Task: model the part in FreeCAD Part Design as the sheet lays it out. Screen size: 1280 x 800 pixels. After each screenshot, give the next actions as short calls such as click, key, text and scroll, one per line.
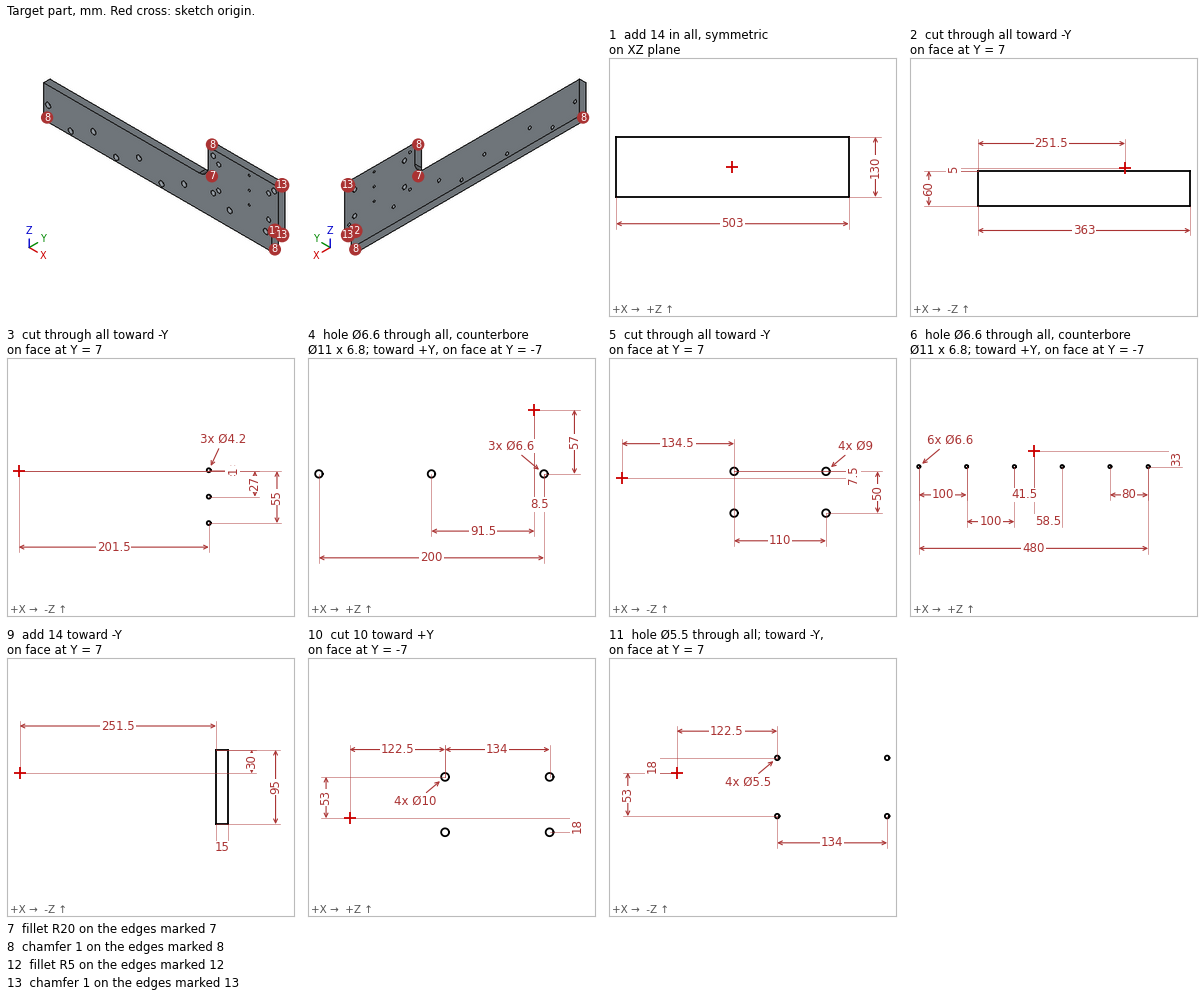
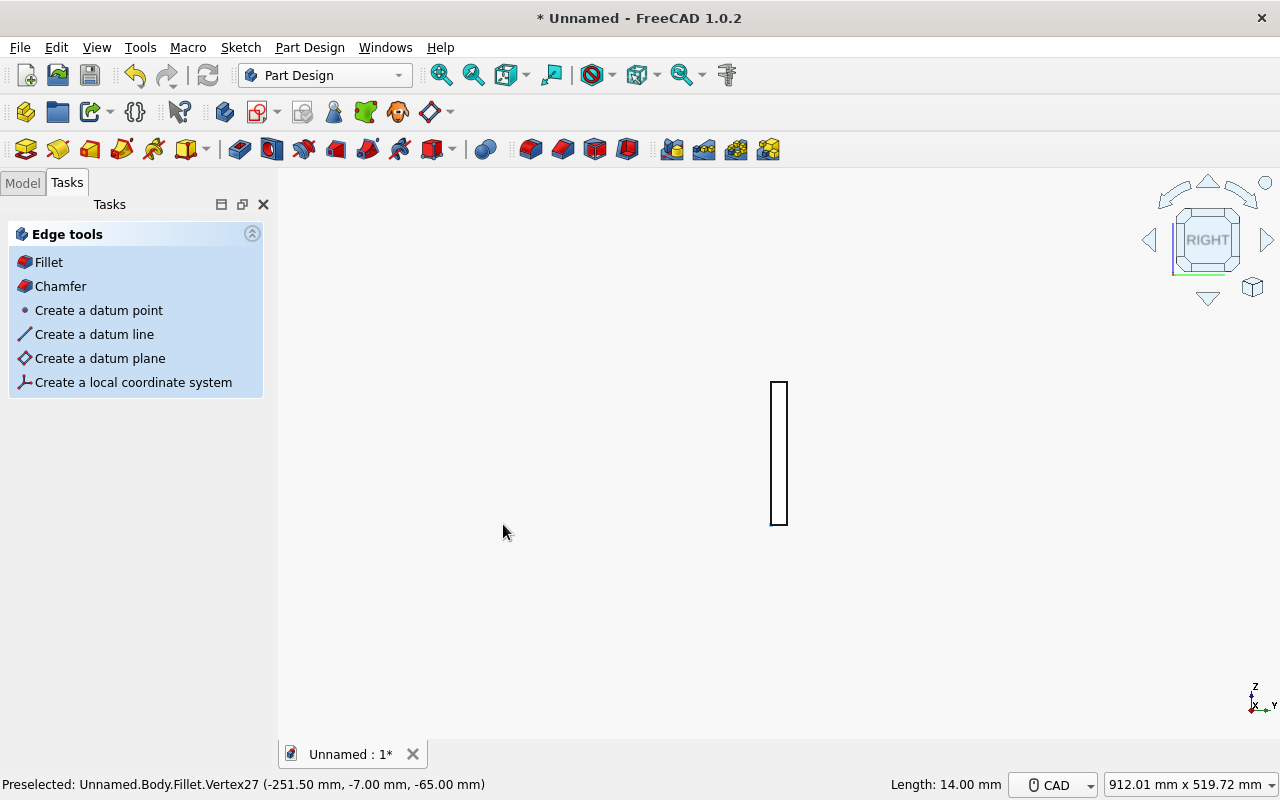
click(442, 76)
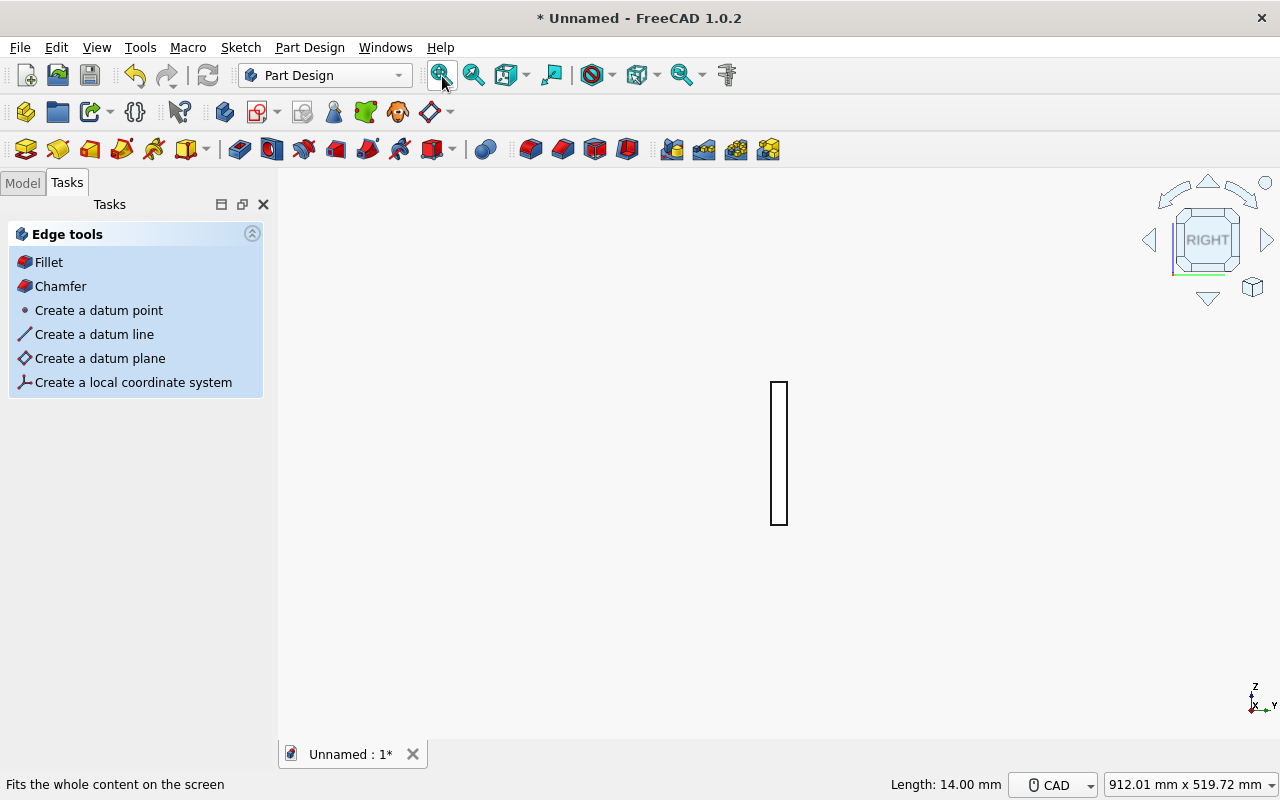
click(779, 524, ctrl)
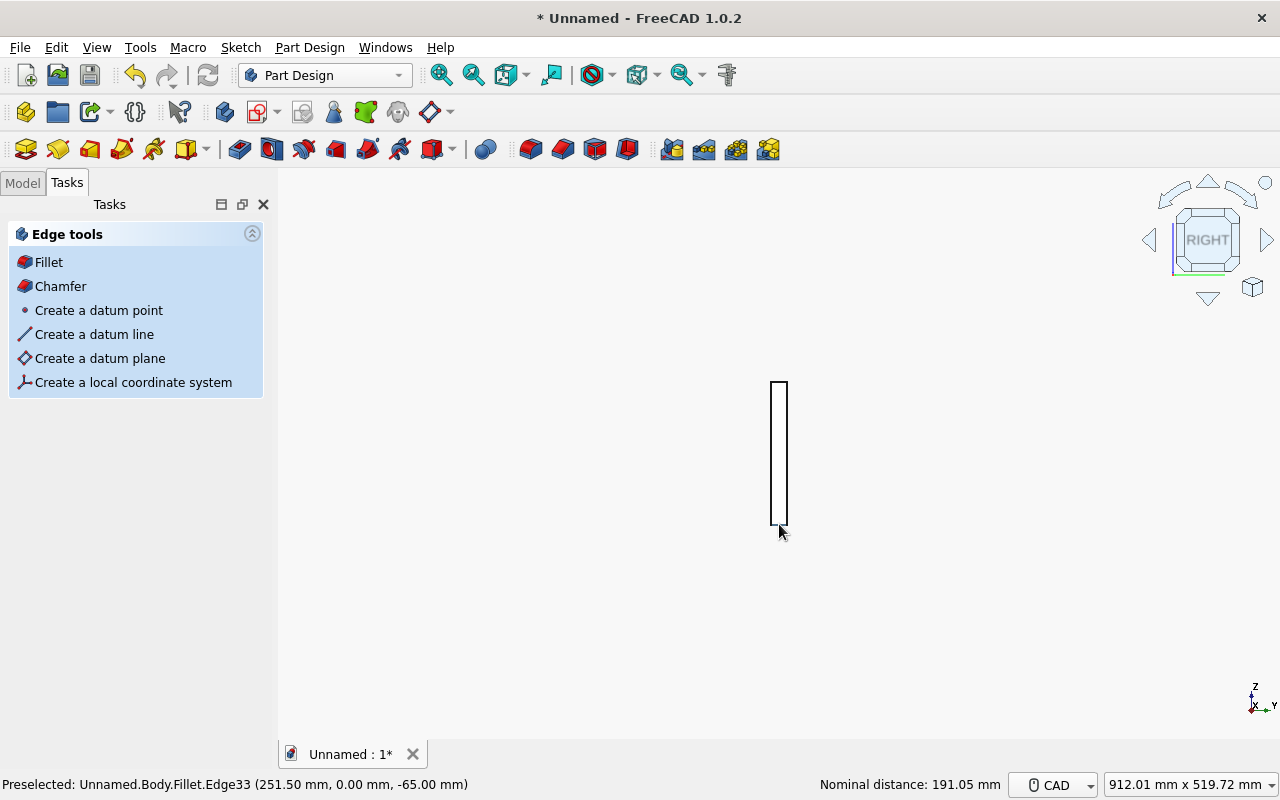
scroll(779, 524, up, 5)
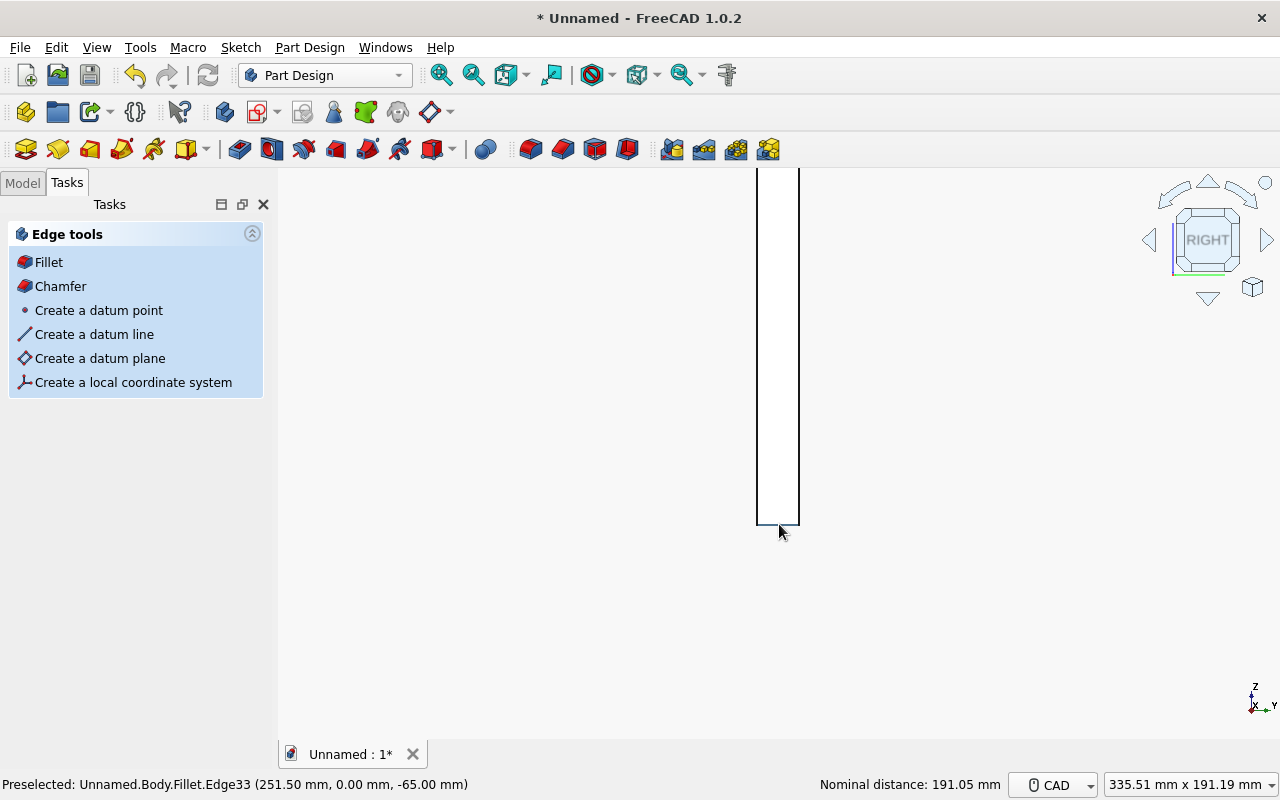
key(v)
key(f)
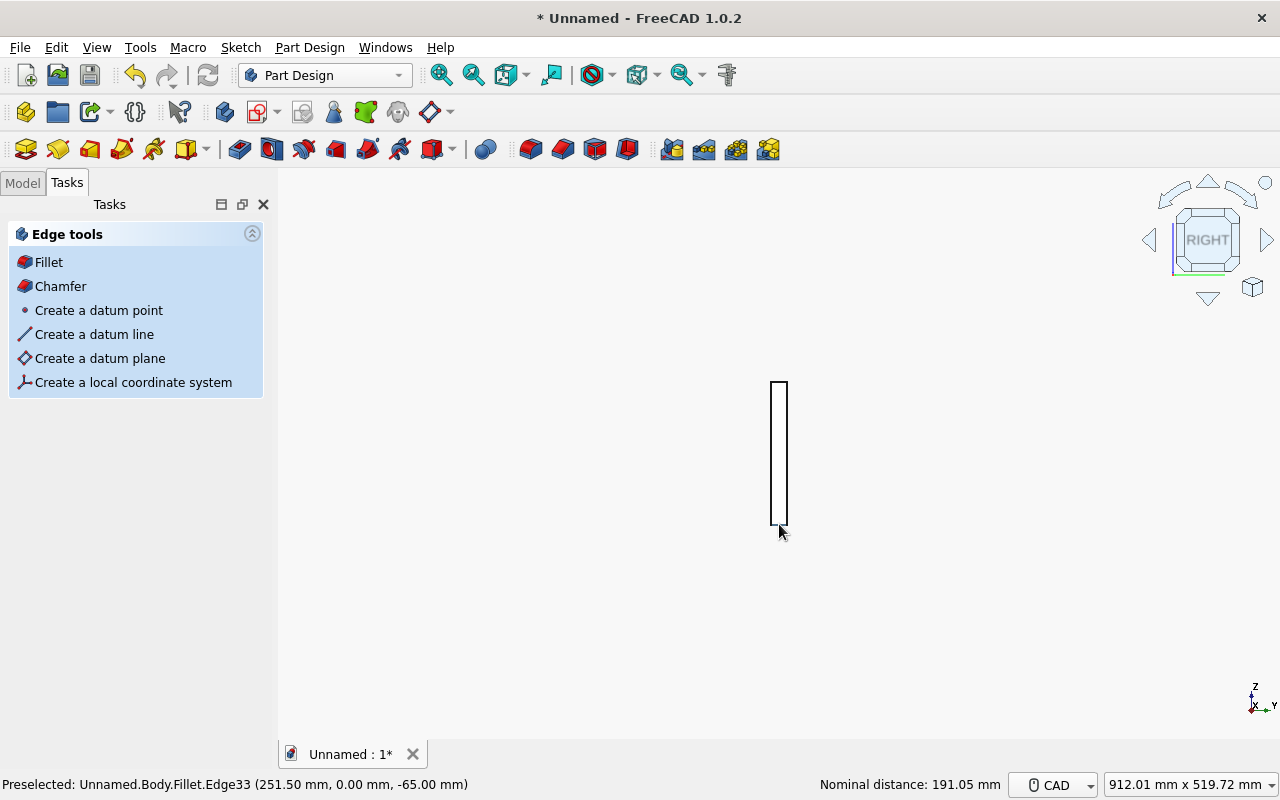
key(5)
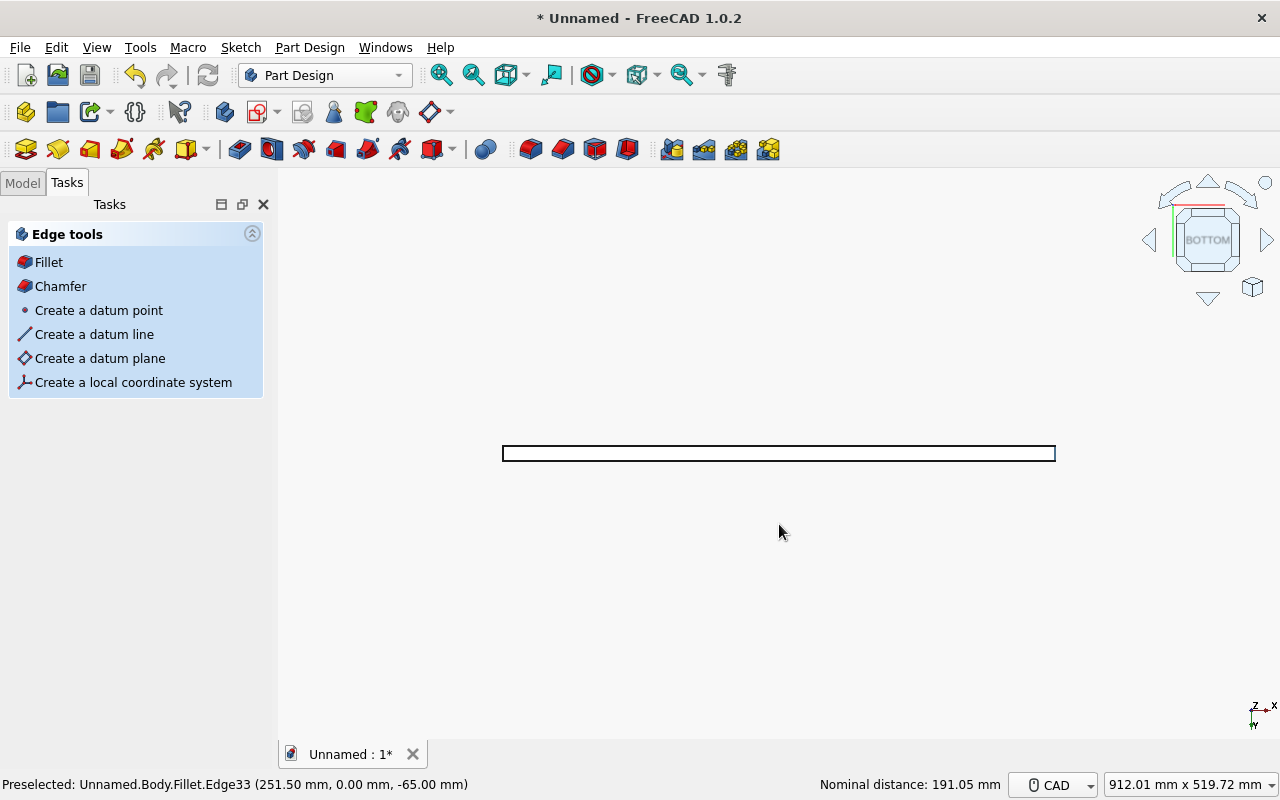
click(503, 452, ctrl)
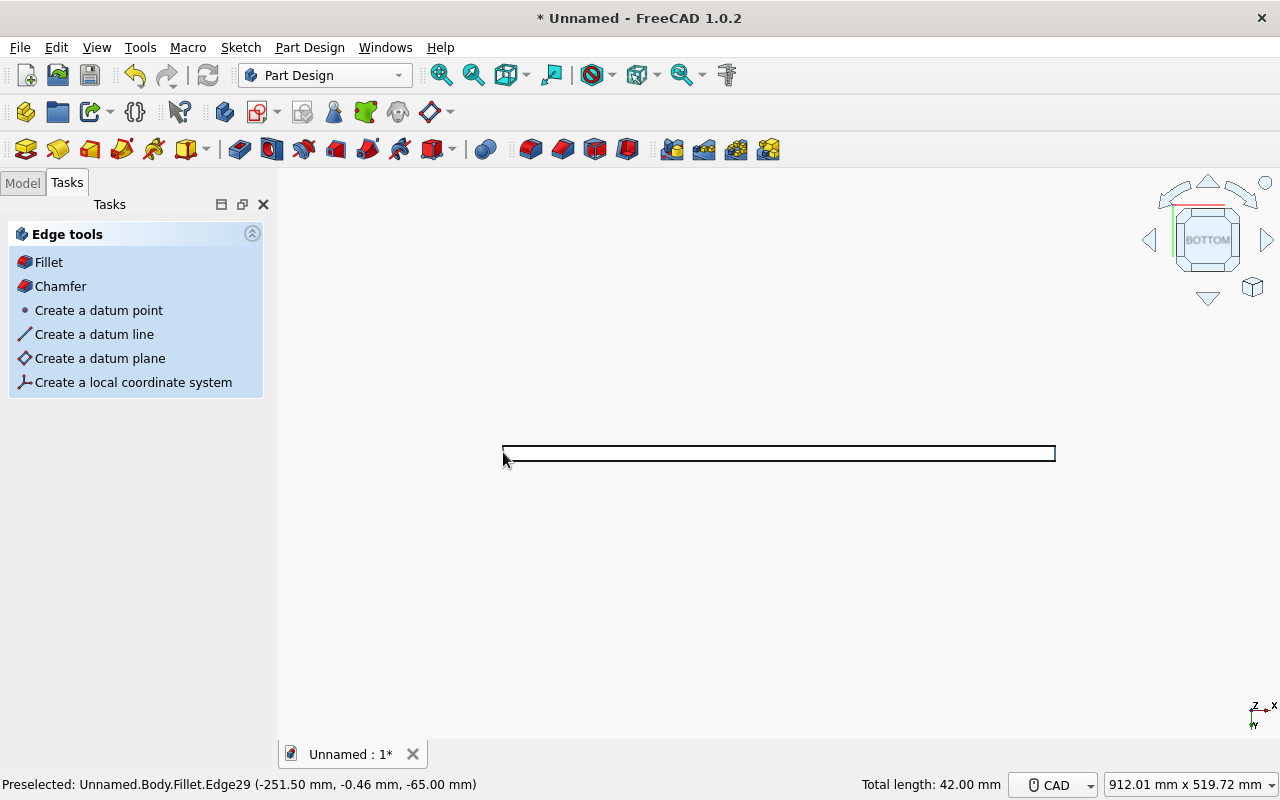
click(564, 150)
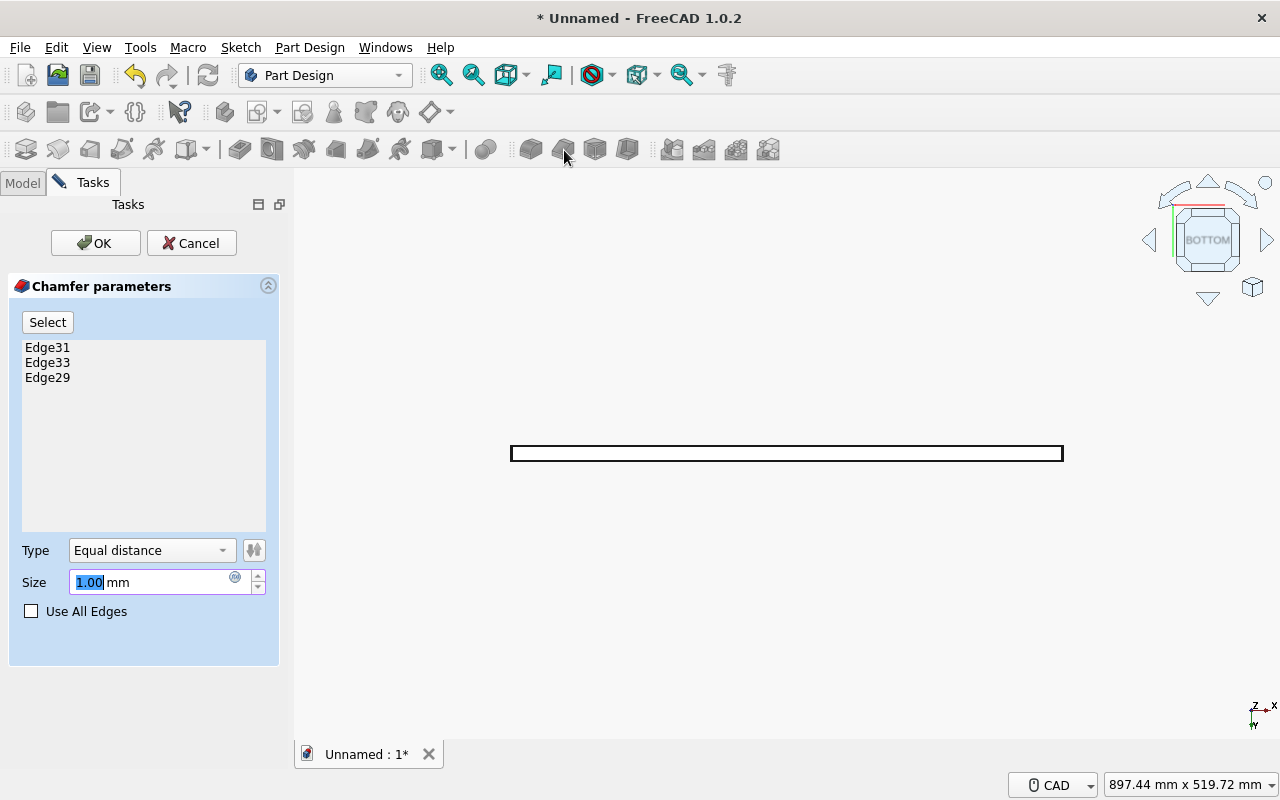
text(1)
key(Tab)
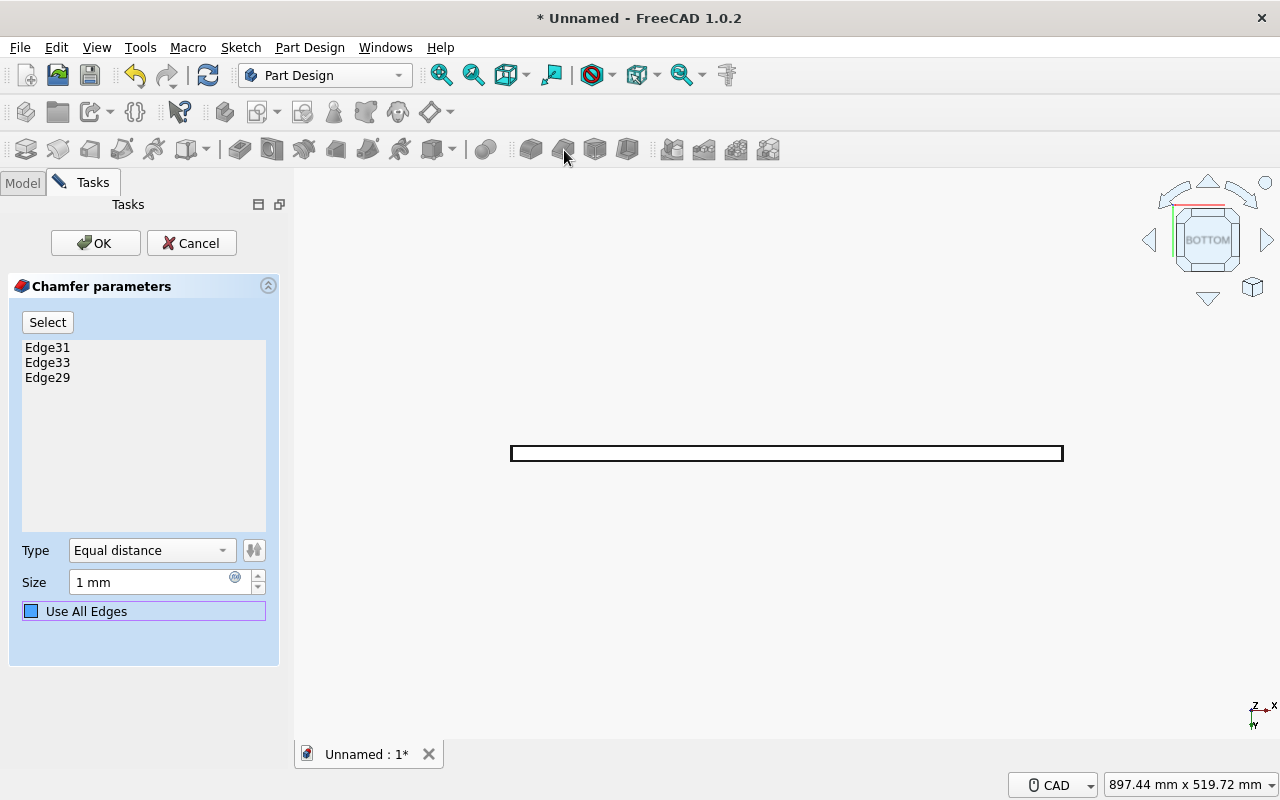
click(96, 243)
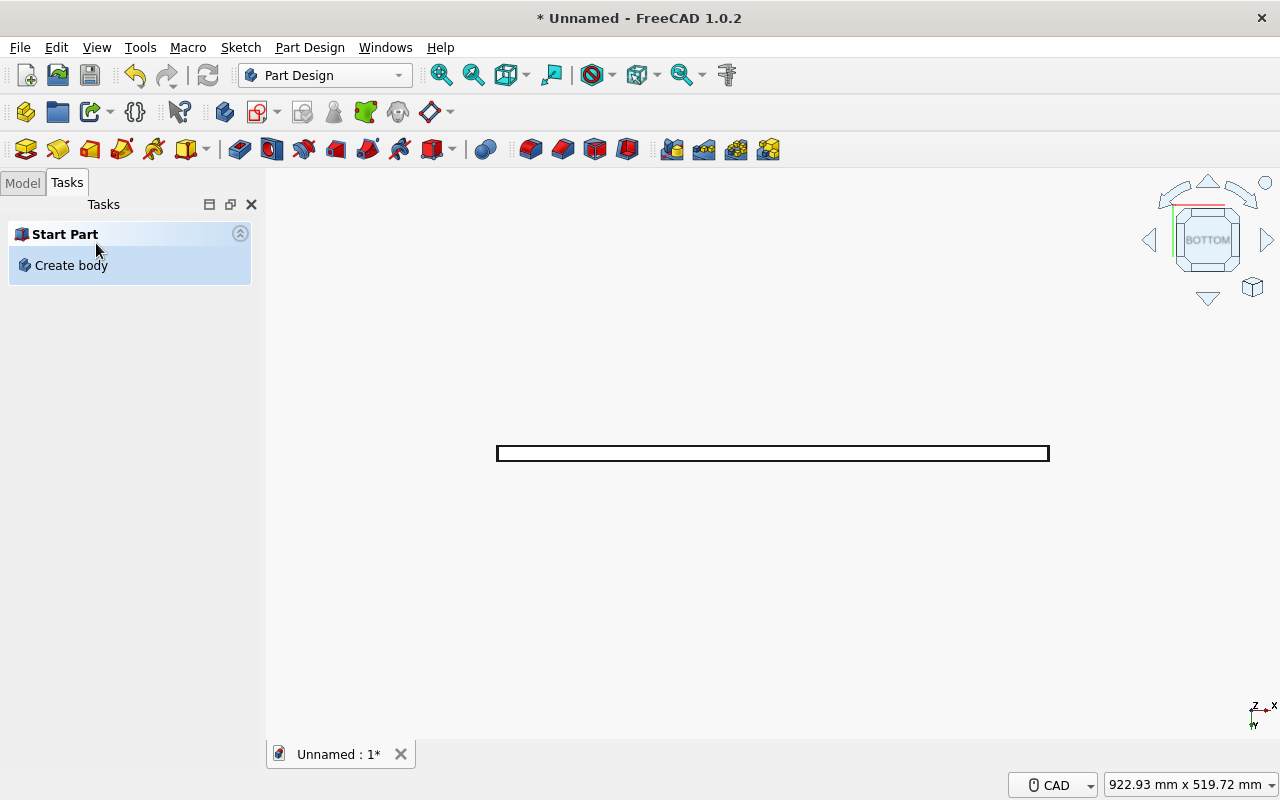
key(4)